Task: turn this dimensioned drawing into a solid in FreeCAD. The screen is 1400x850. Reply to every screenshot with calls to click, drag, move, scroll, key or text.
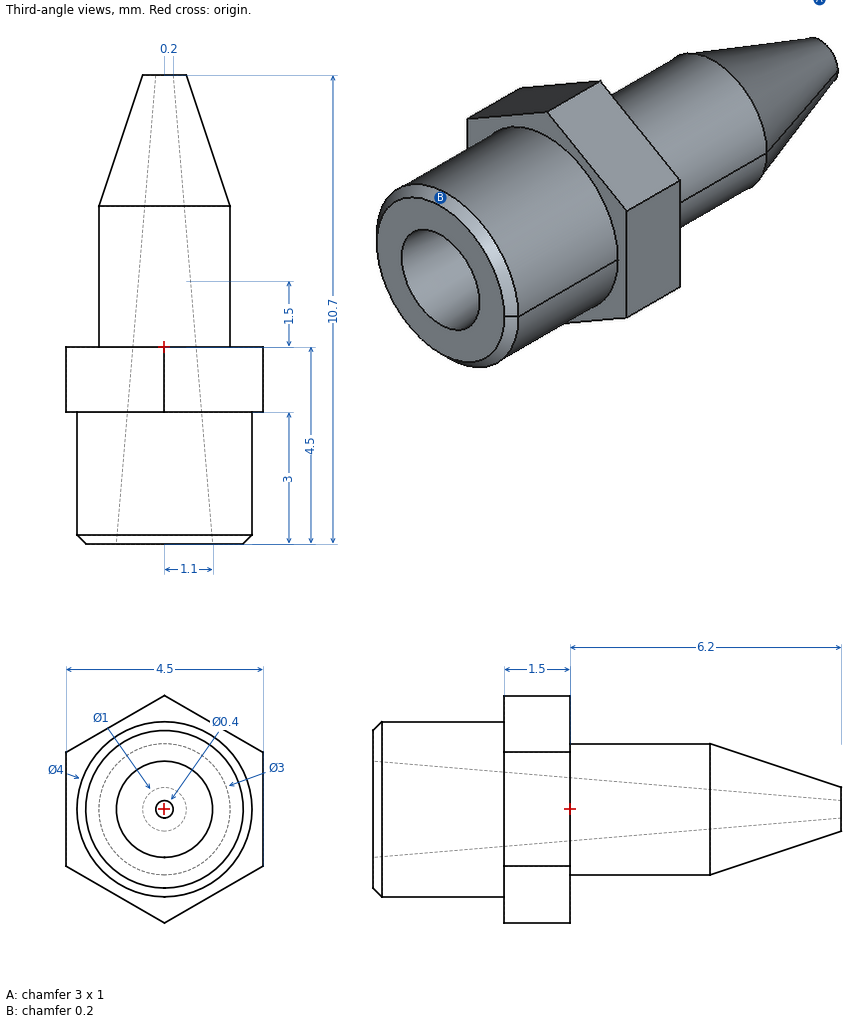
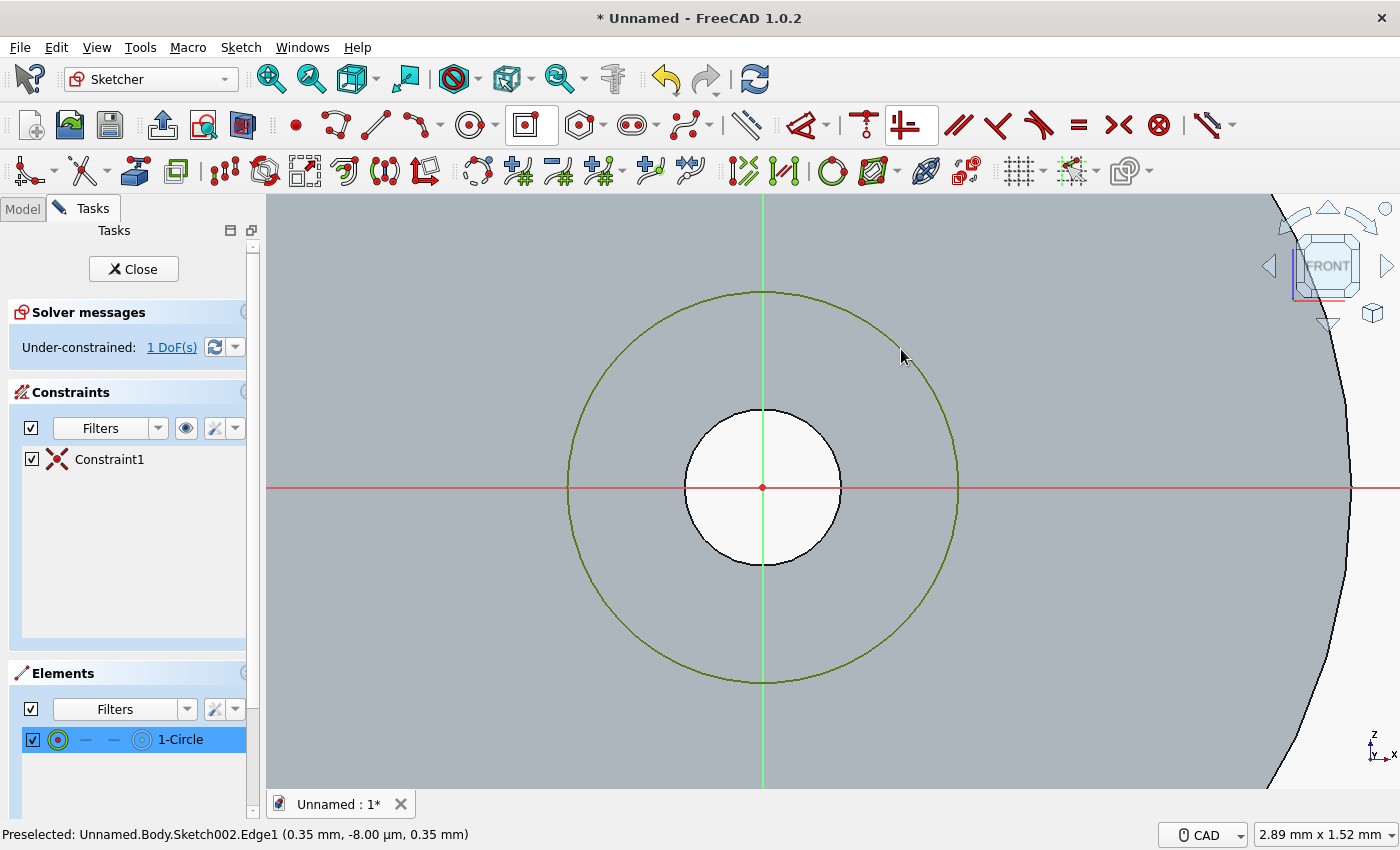
click(828, 126)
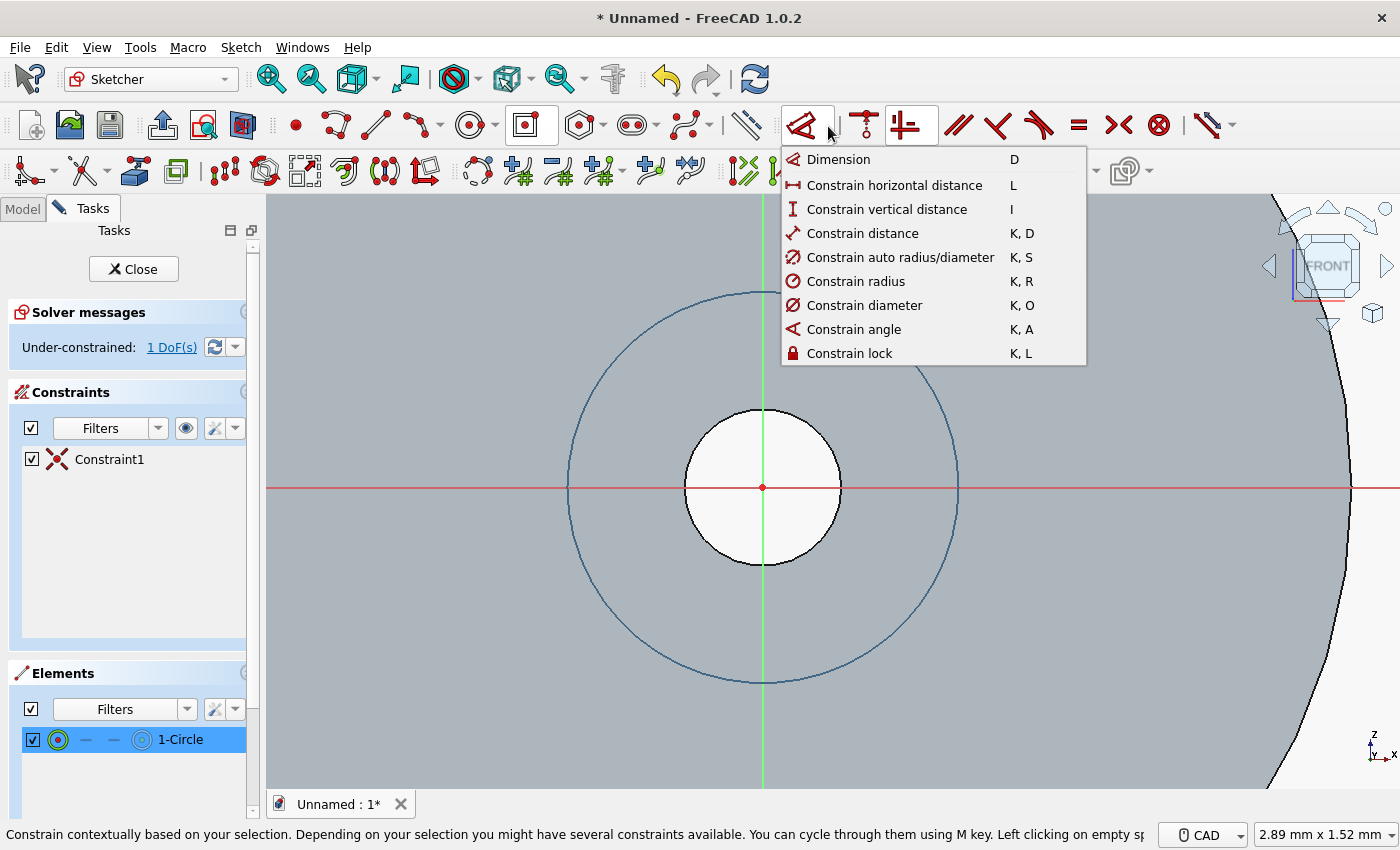
click(934, 305)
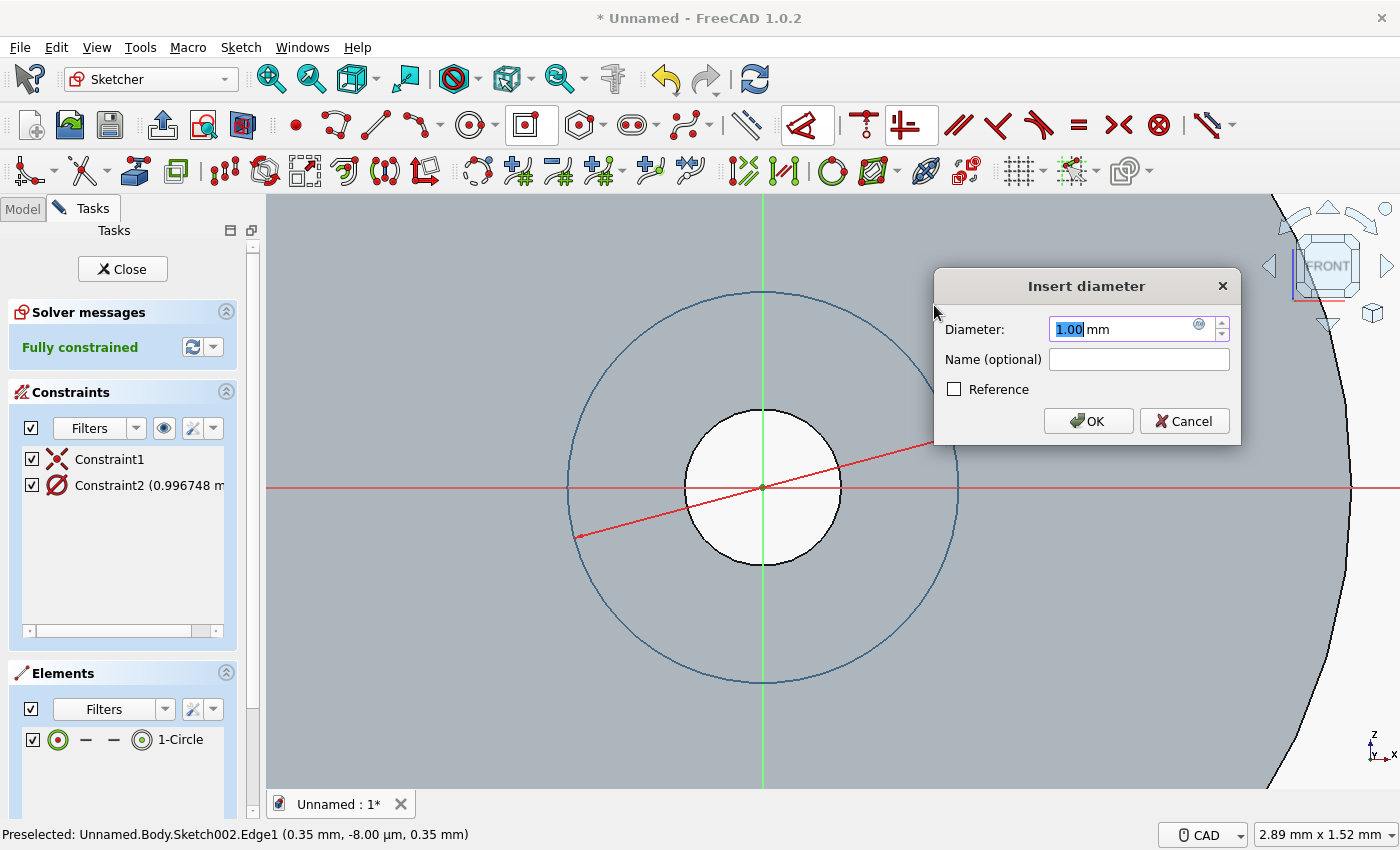
text(1)
key(Return)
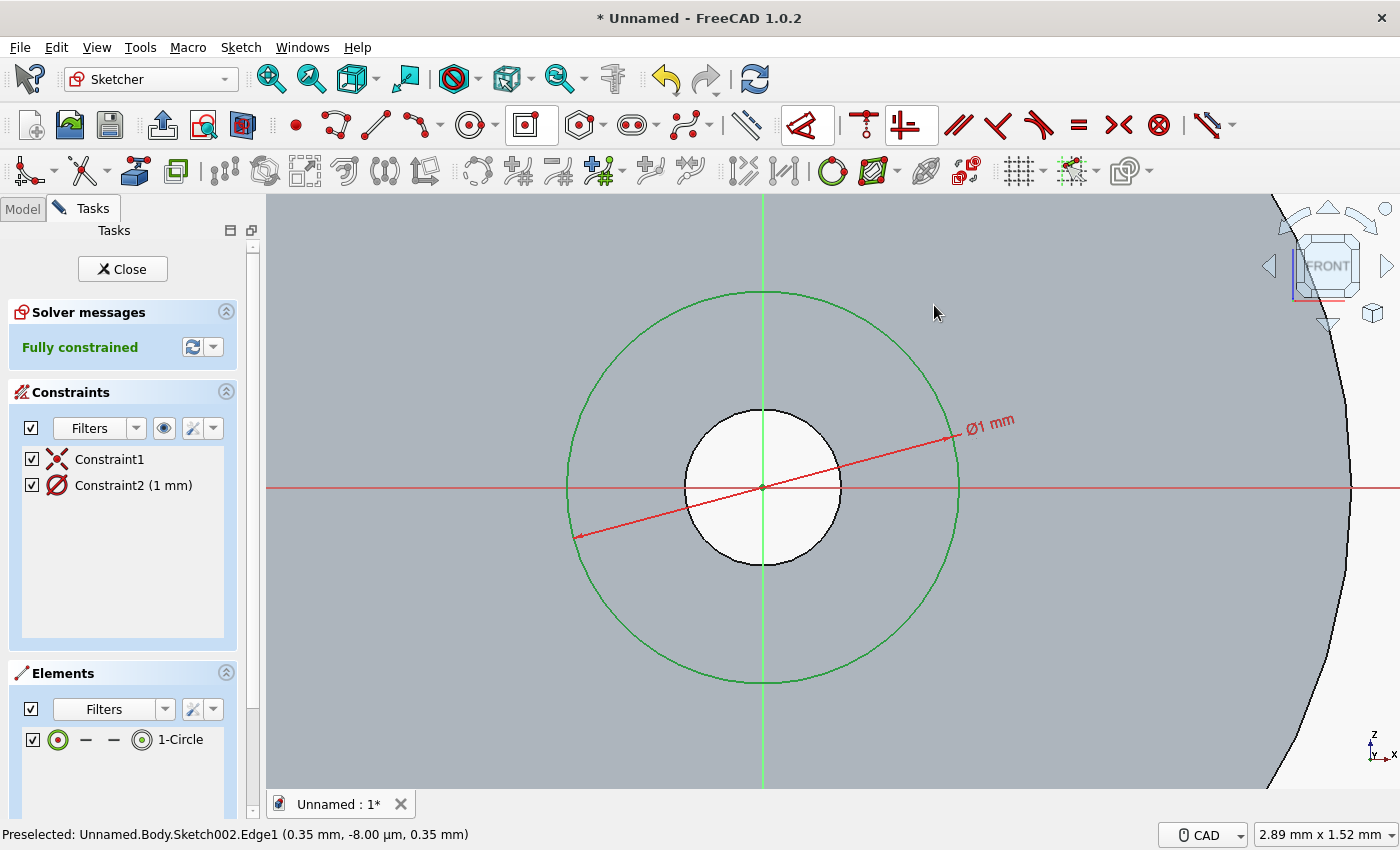
click(123, 269)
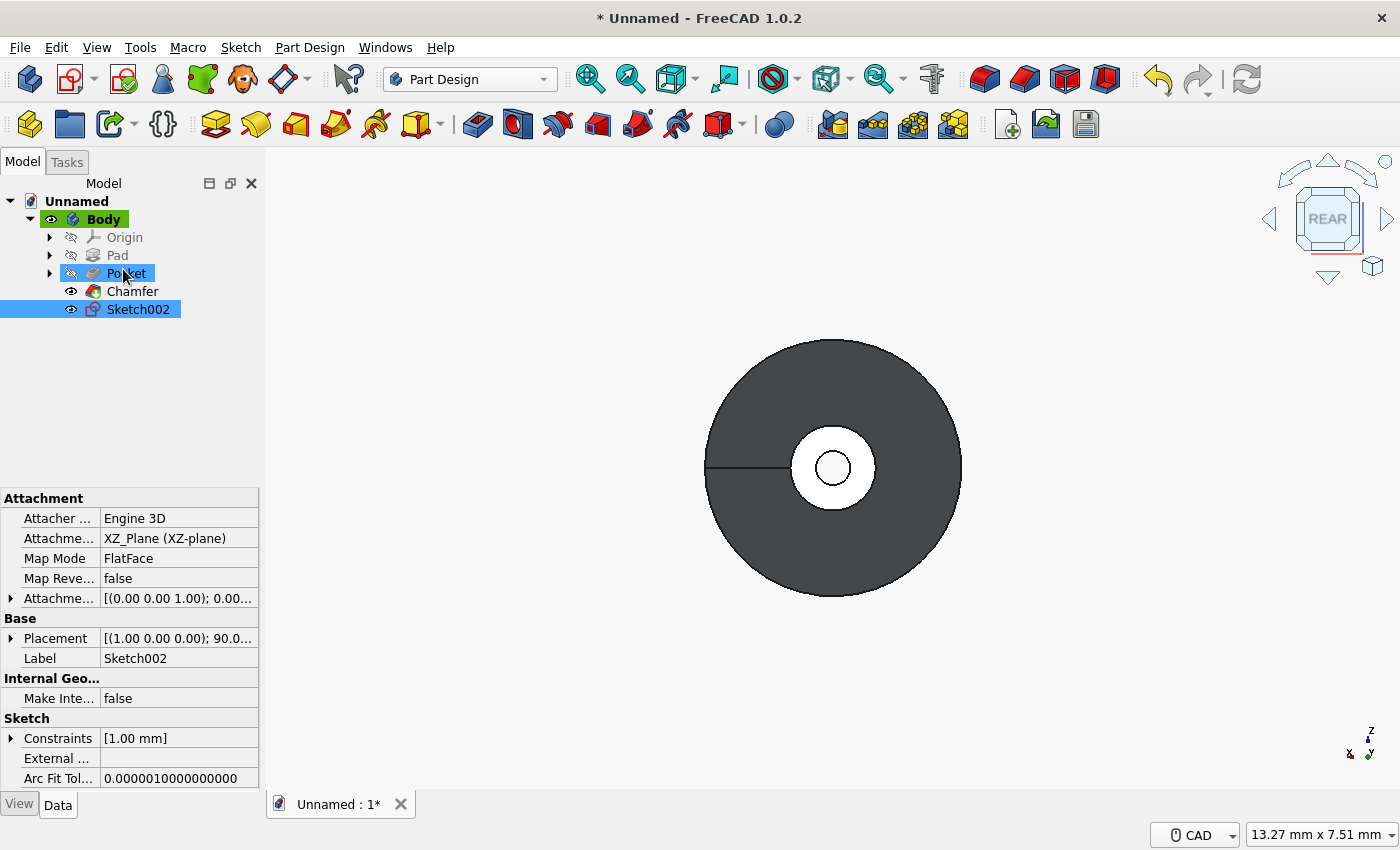
click(478, 124)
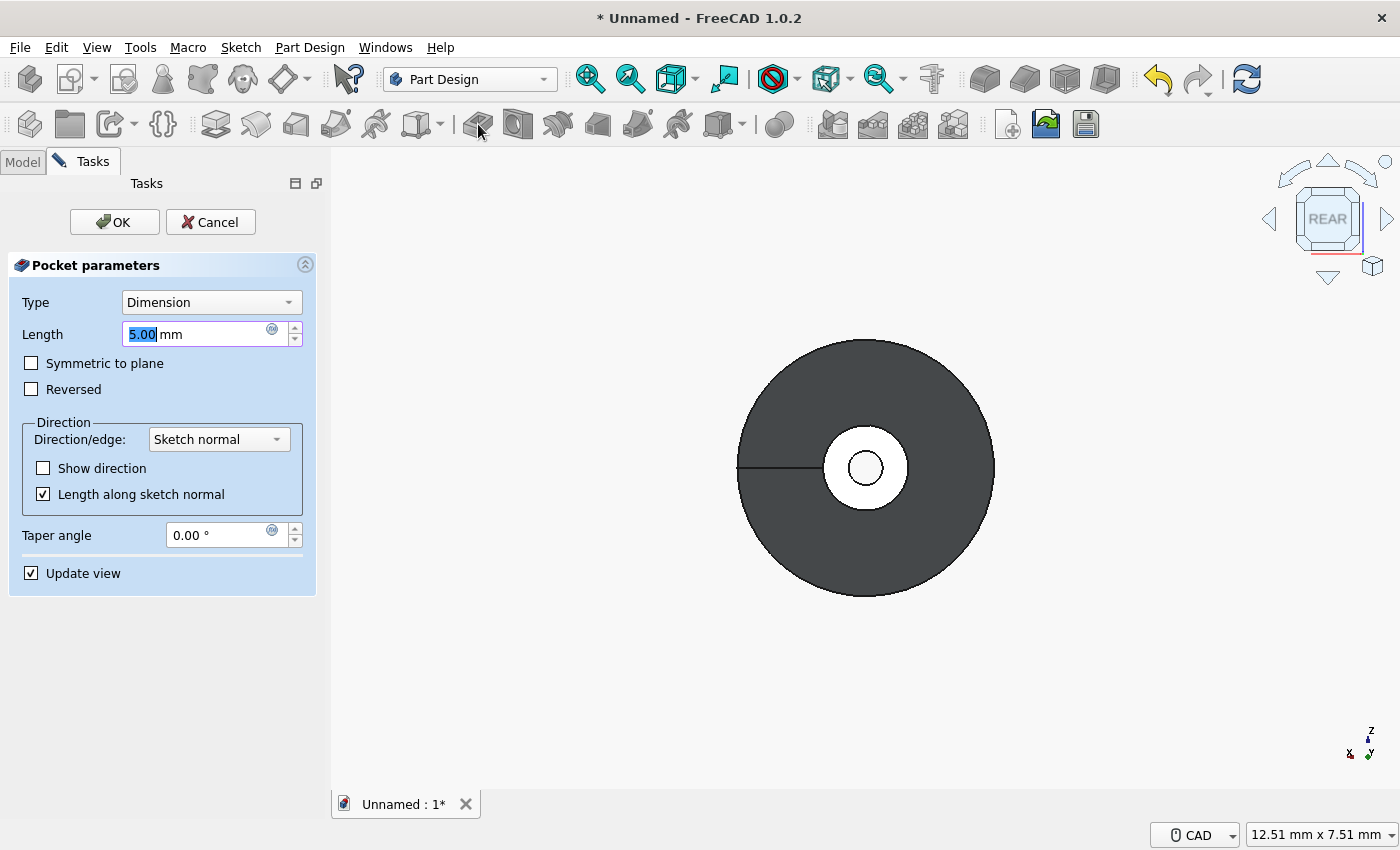
text(1.5)
key(Tab)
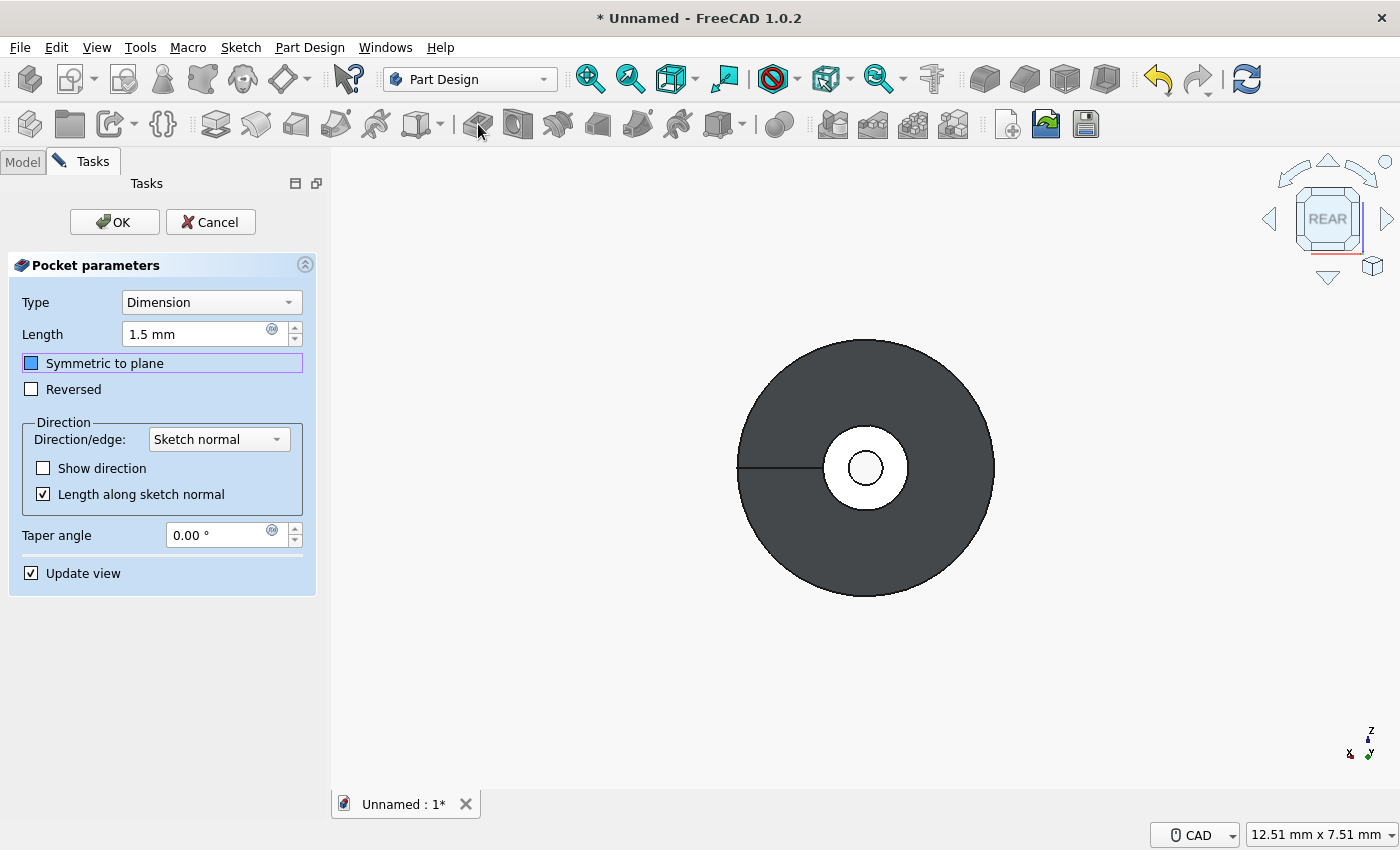
click(115, 222)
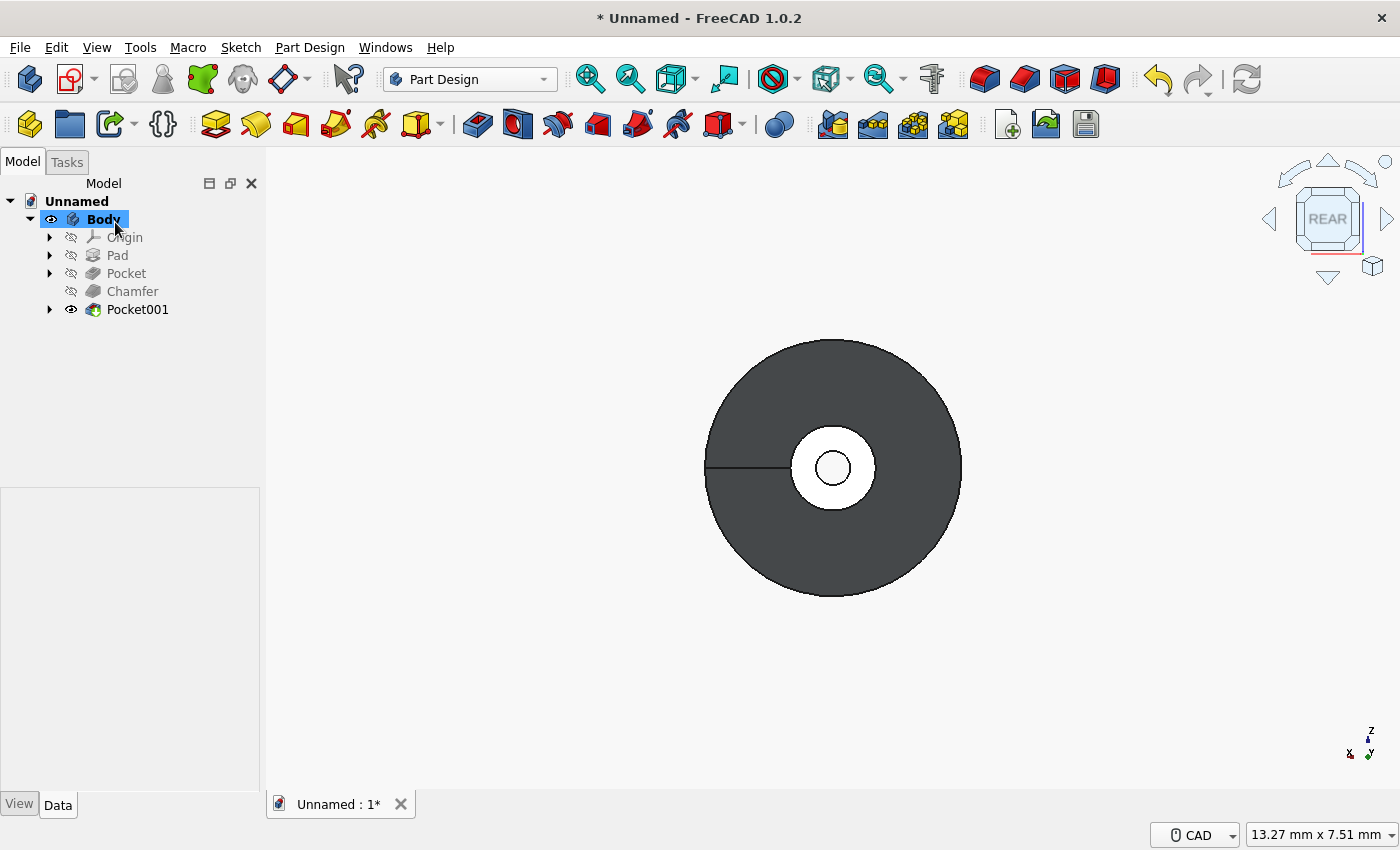
click(592, 80)